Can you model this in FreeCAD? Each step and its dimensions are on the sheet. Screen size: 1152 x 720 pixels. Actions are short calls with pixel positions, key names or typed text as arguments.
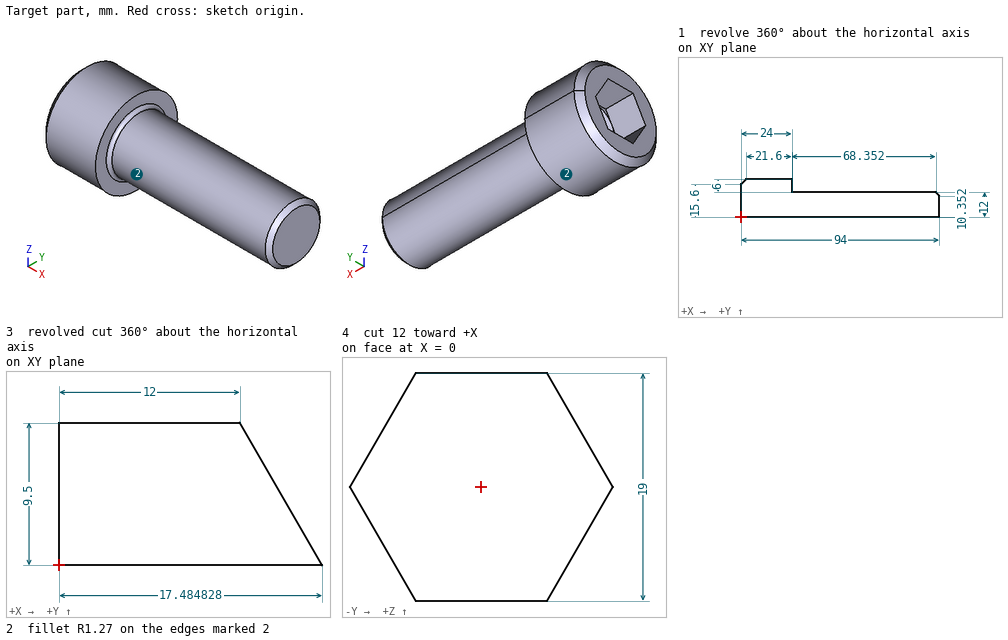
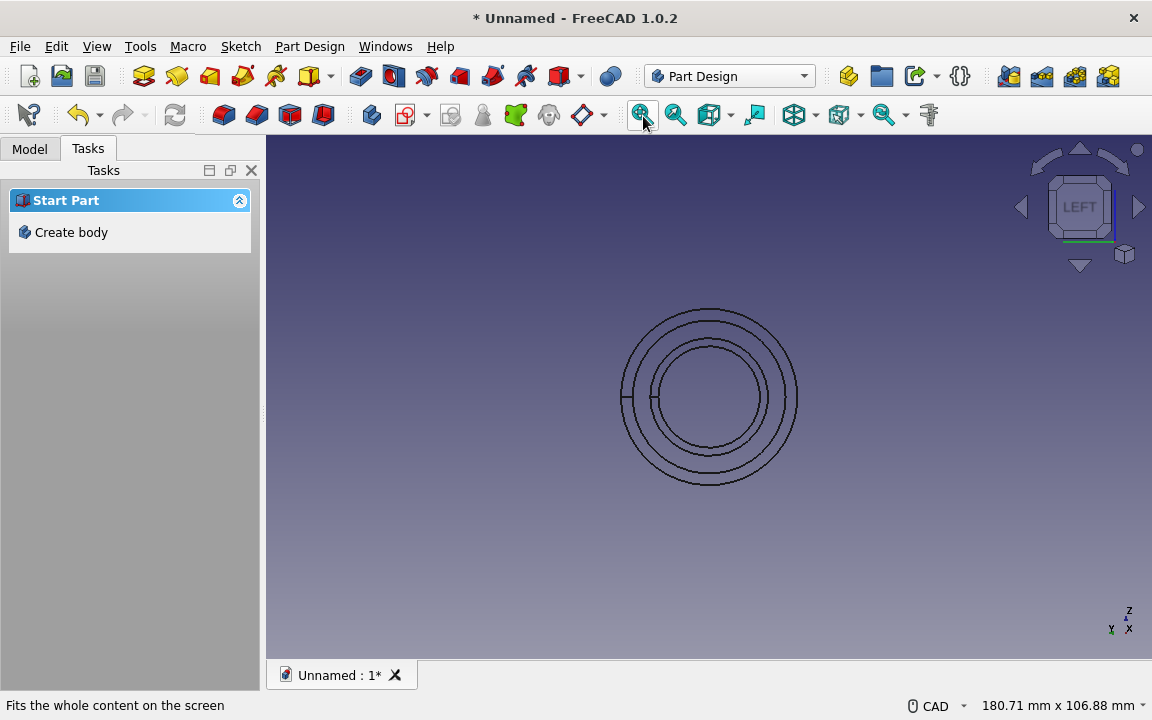
key(0)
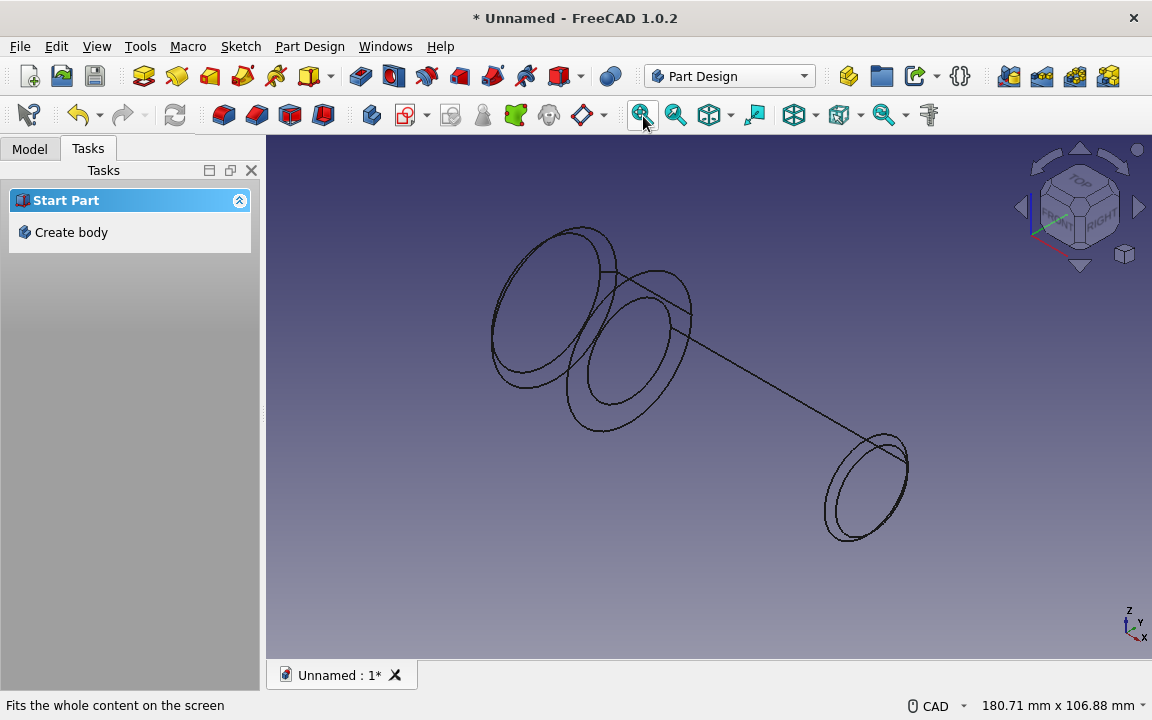
click(588, 374)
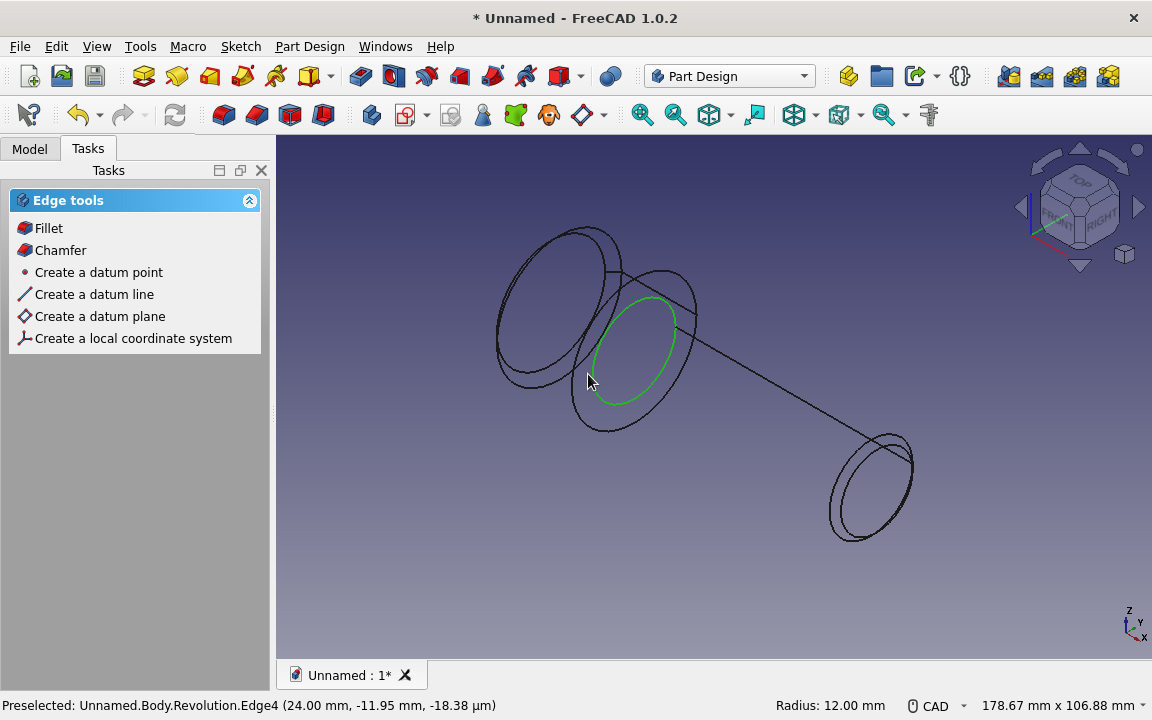
key(v)
key(1)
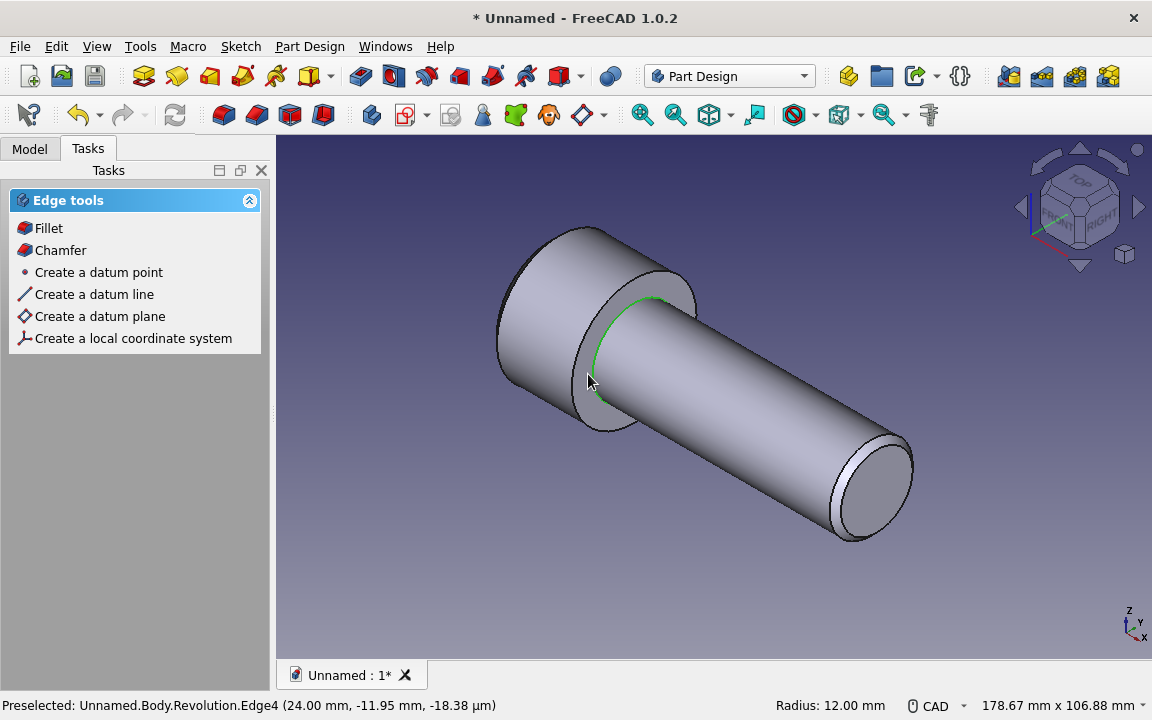
click(224, 116)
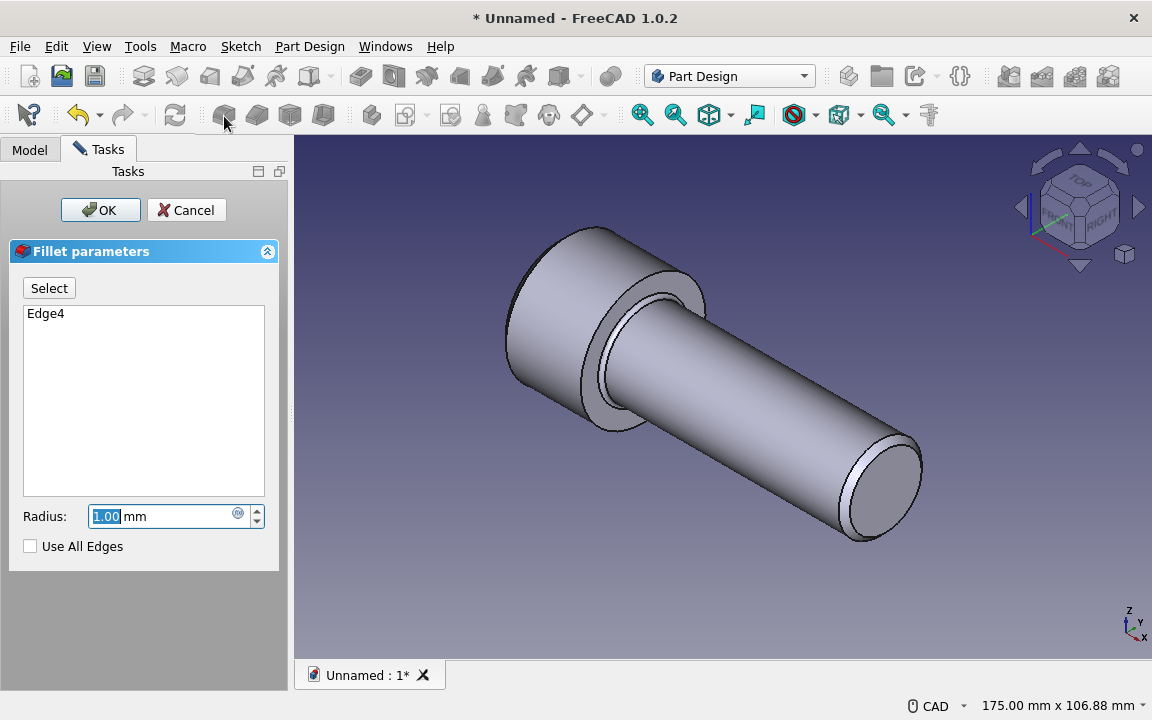
text(1.27)
key(Tab)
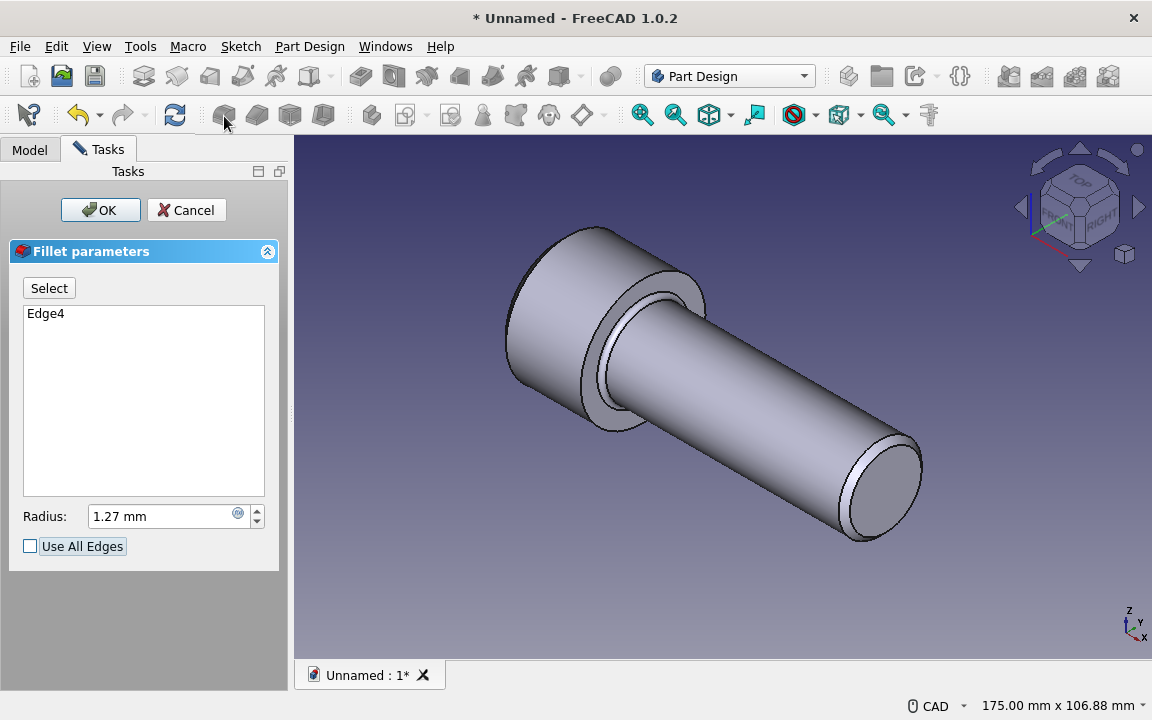
click(101, 210)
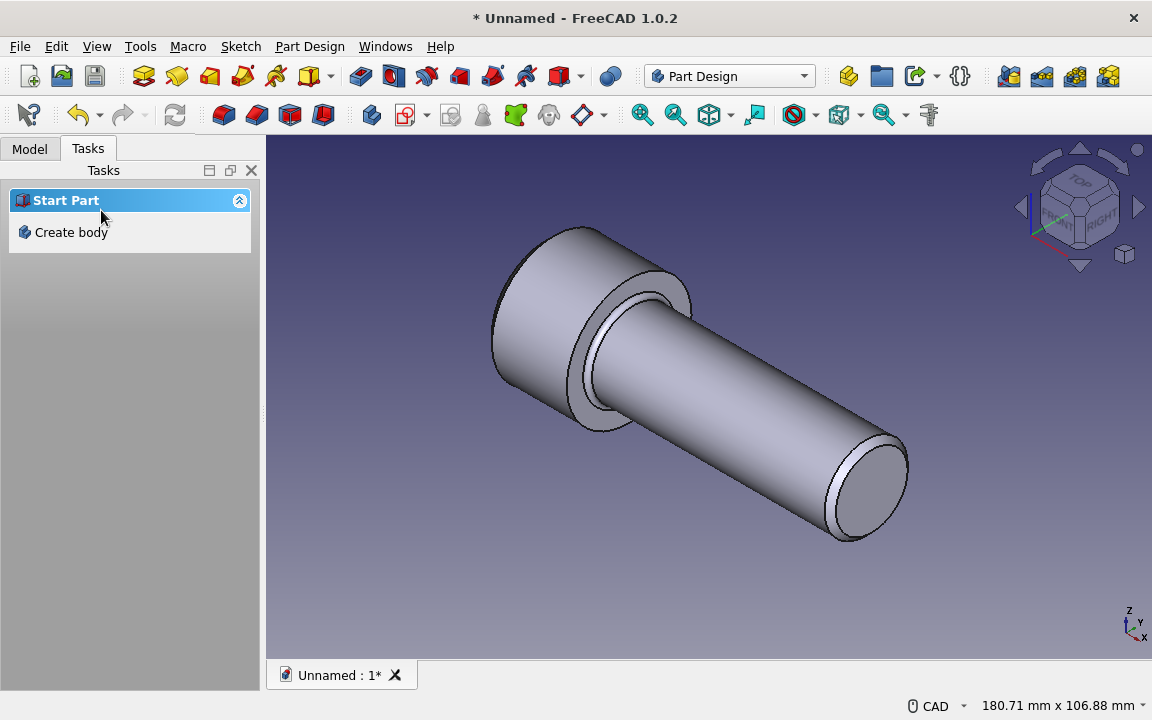
click(404, 116)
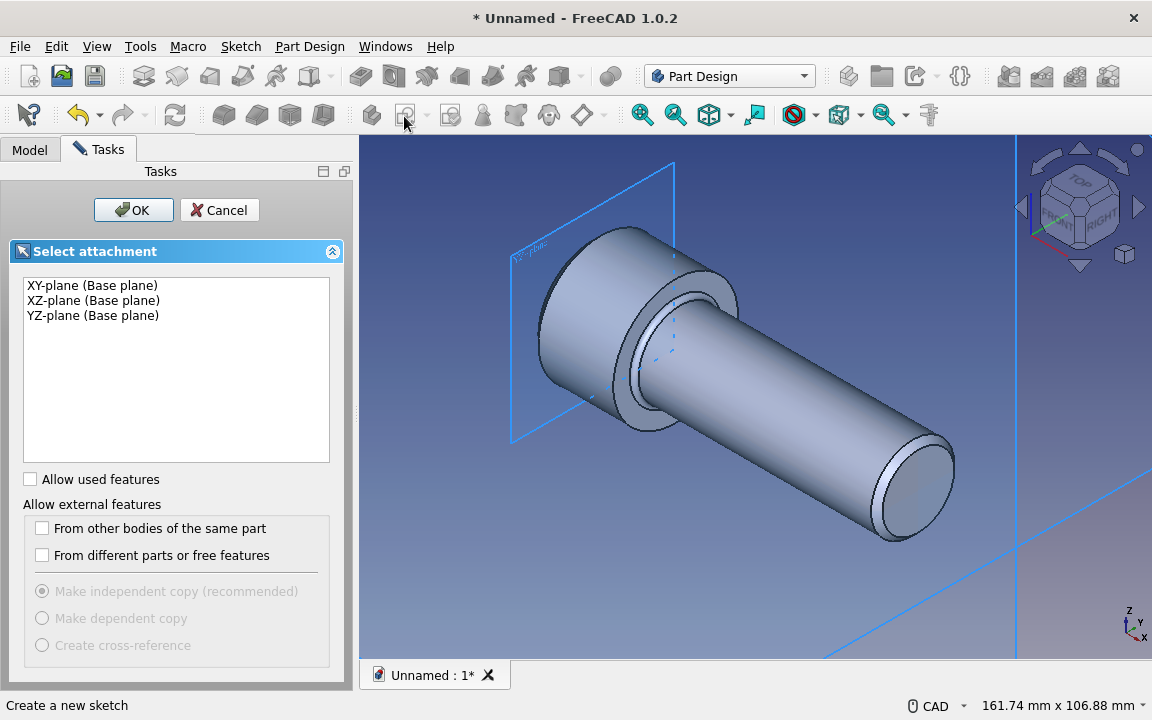
click(84, 286)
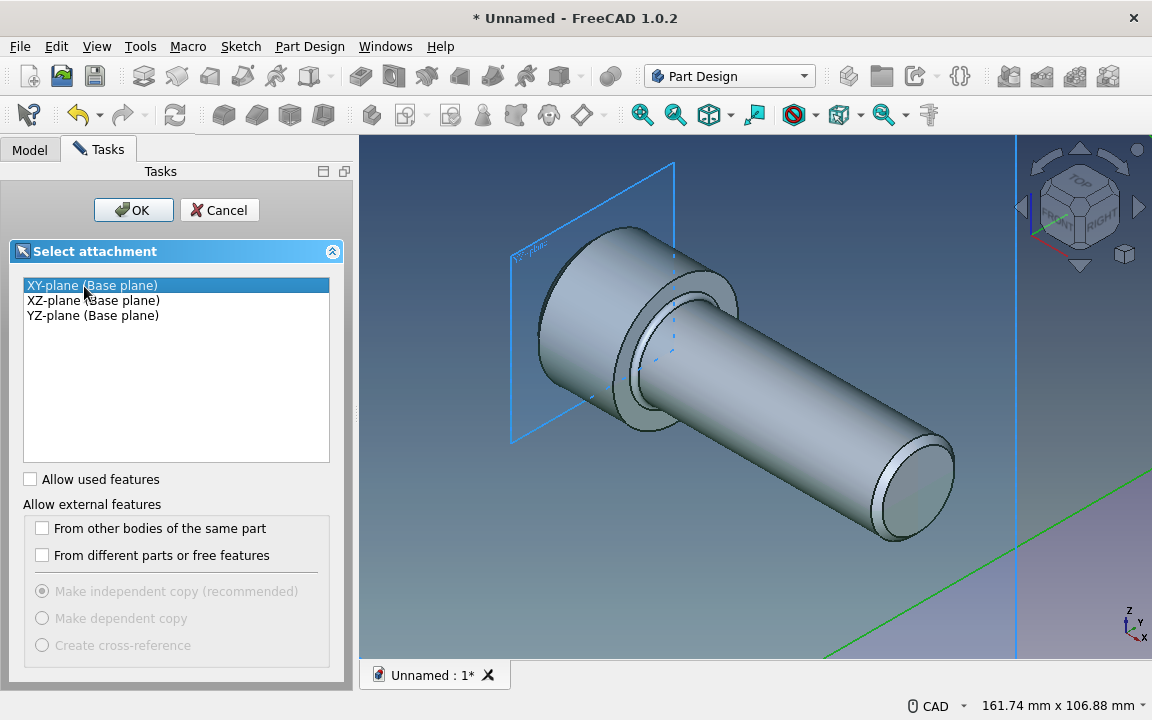
click(134, 210)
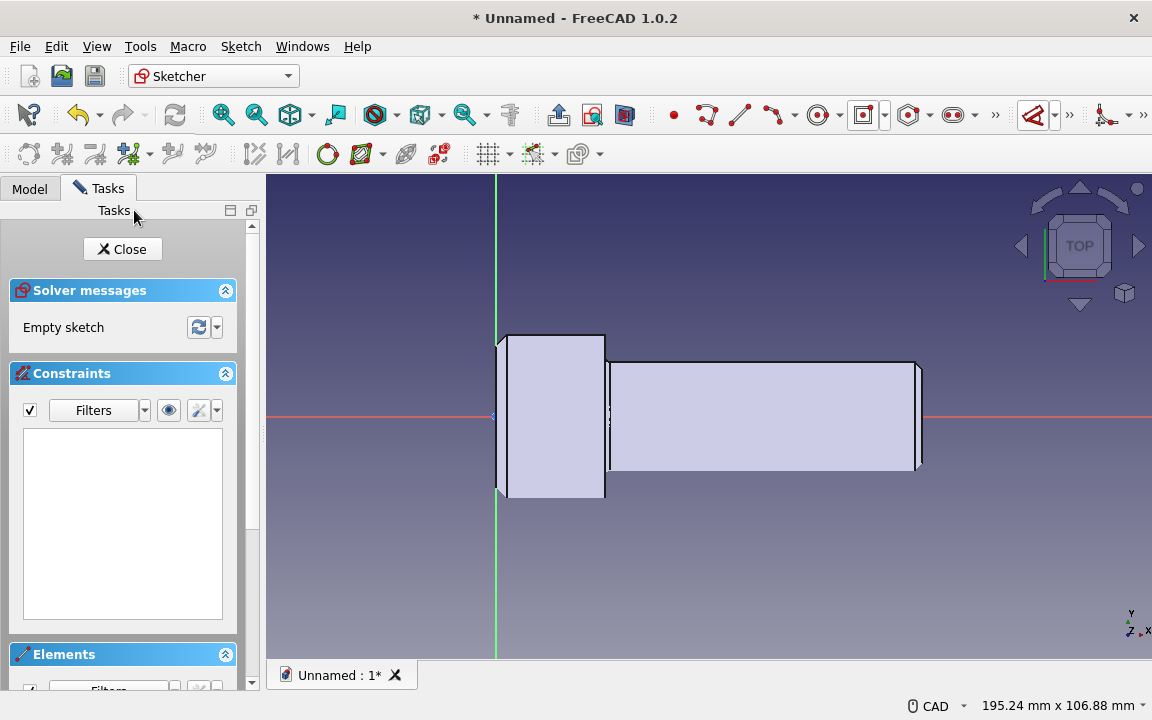
click(625, 116)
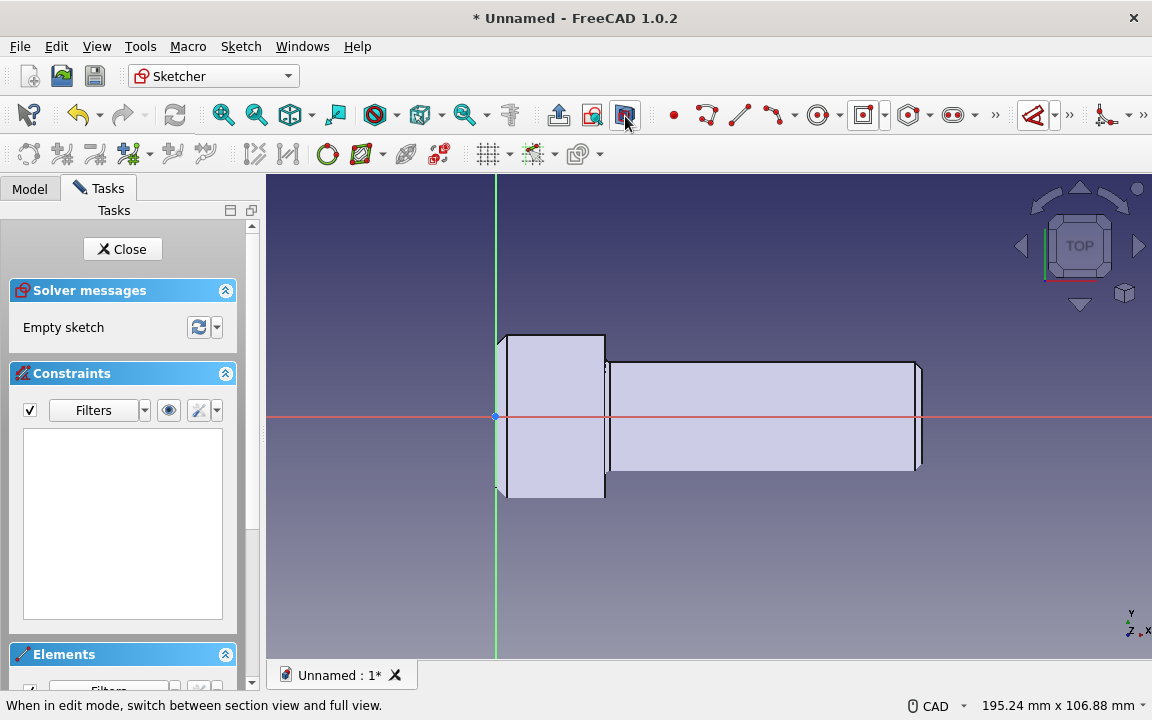
scroll(515, 391, up, 9)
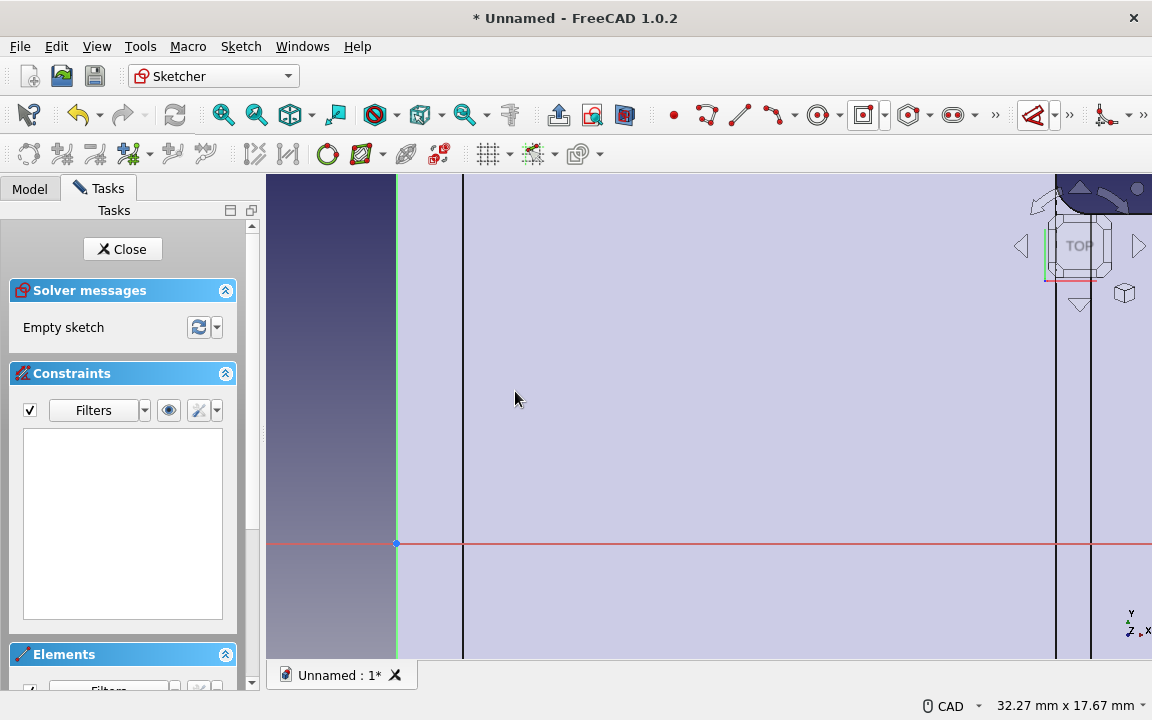
click(707, 116)